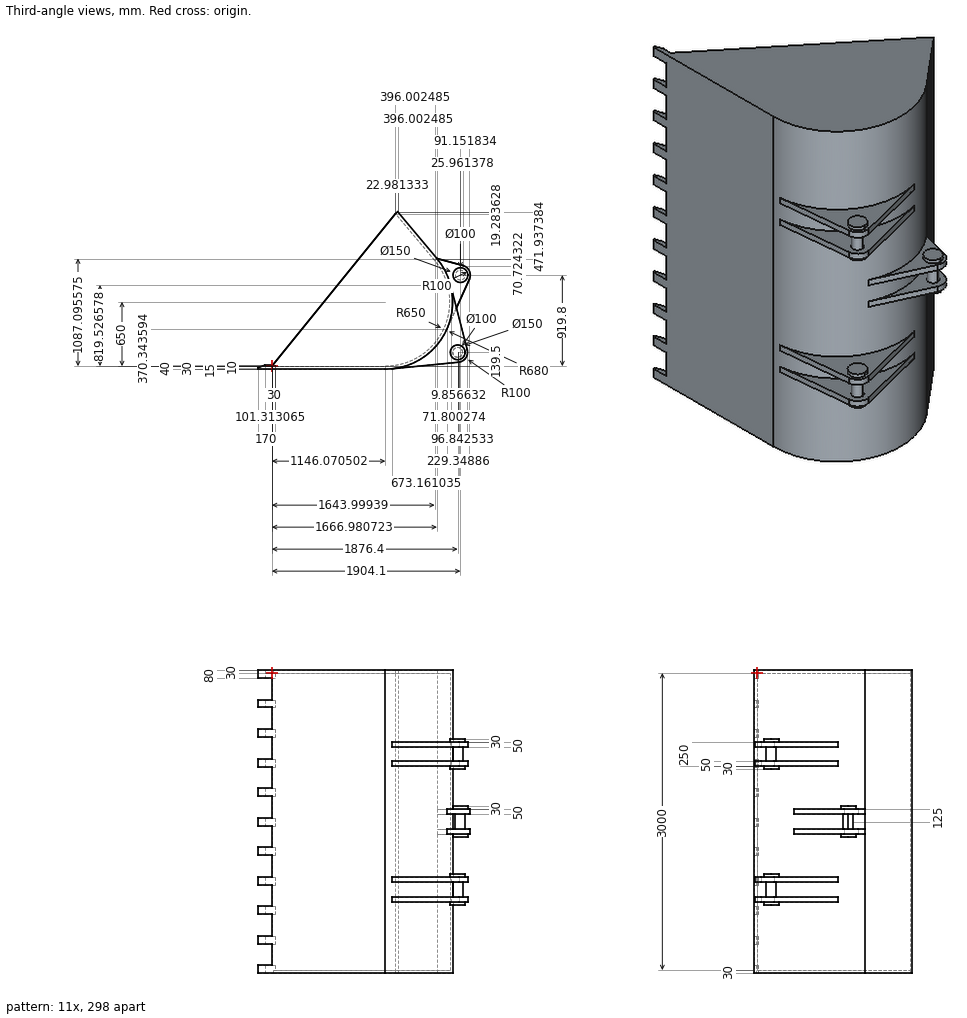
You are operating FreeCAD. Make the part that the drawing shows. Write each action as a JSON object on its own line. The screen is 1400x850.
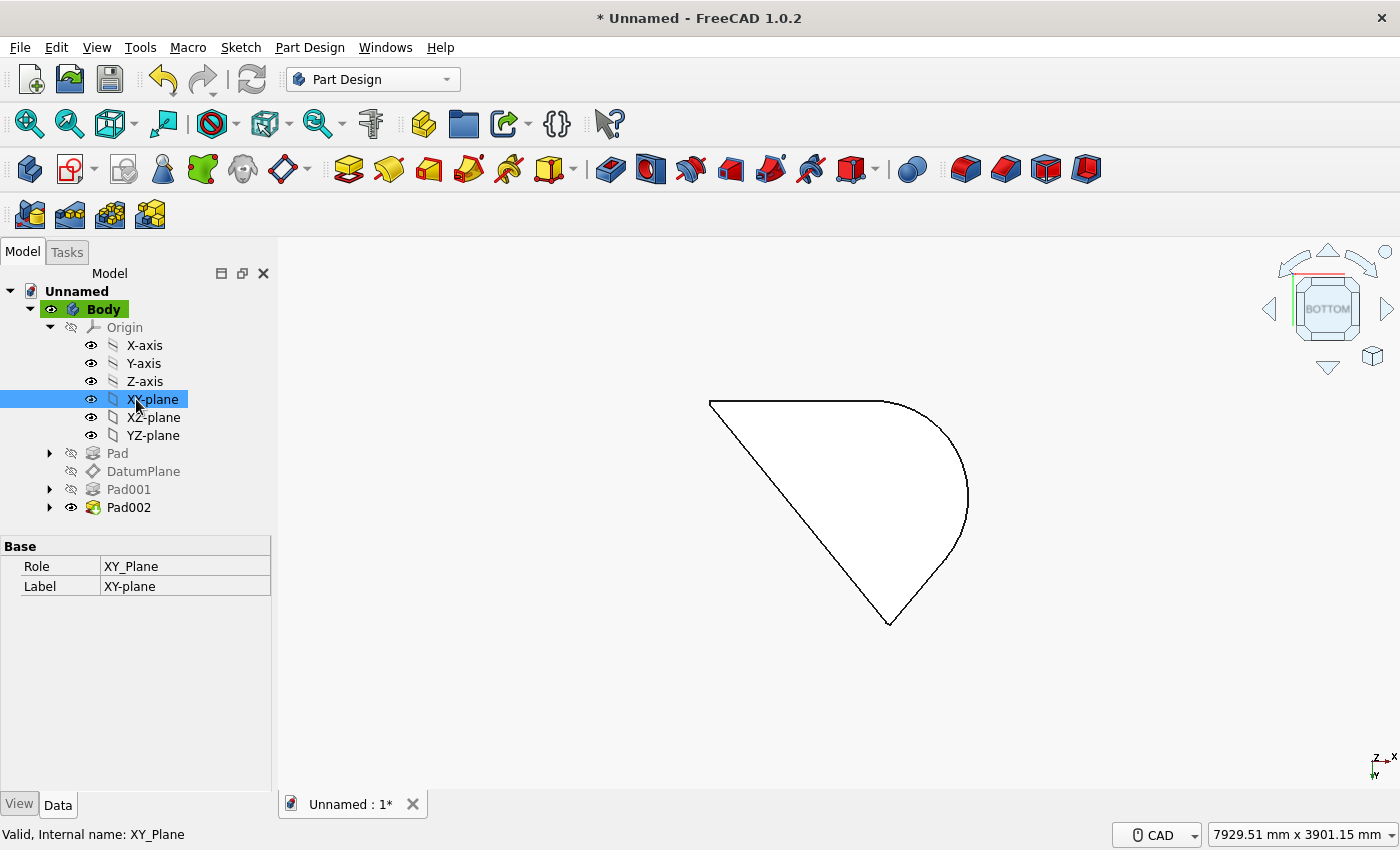
{"action": "left_click", "coordinate": [284, 170]}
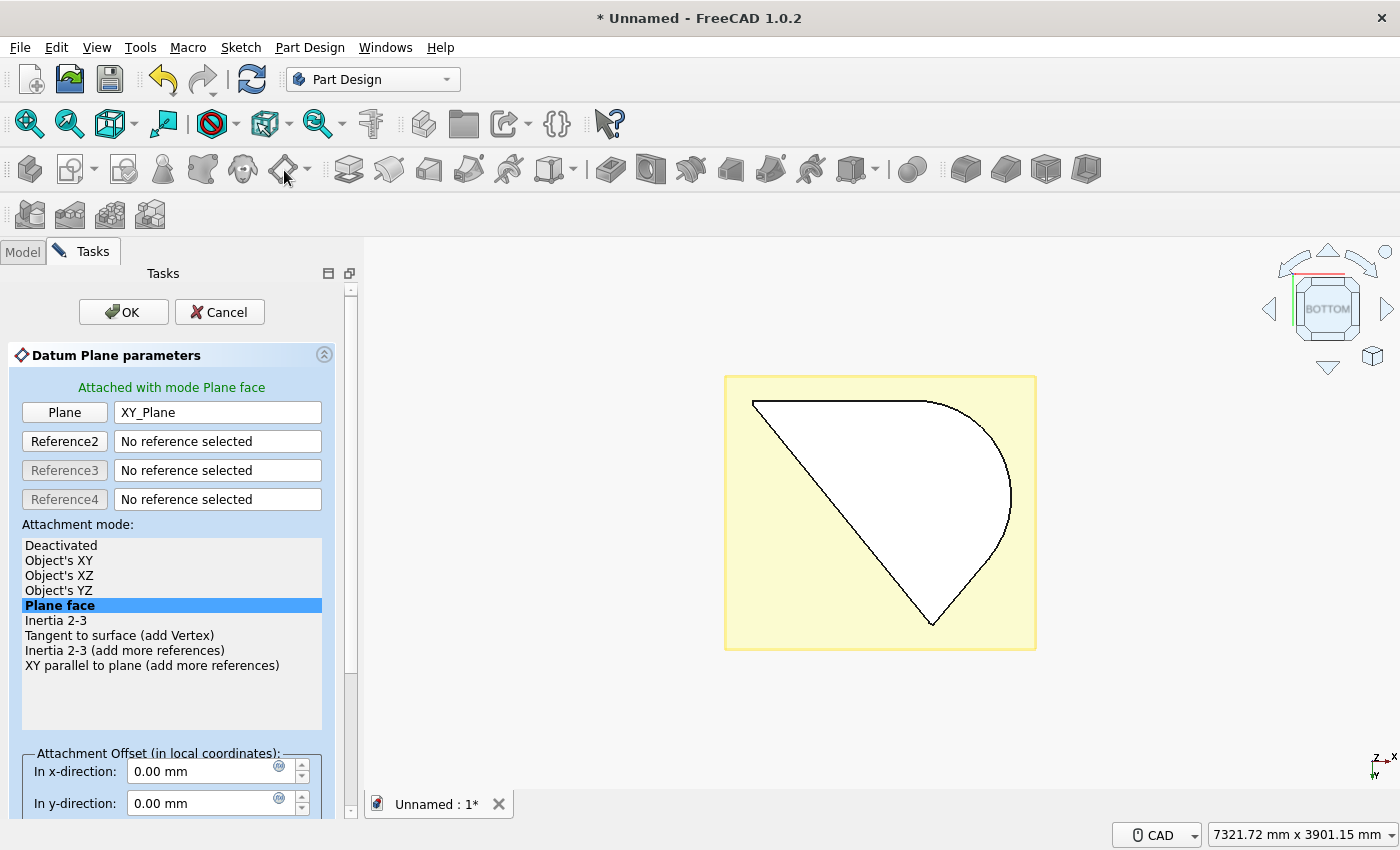
{"action": "scroll", "coordinate": [351, 550], "scroll_direction": "down", "scroll_amount": 2}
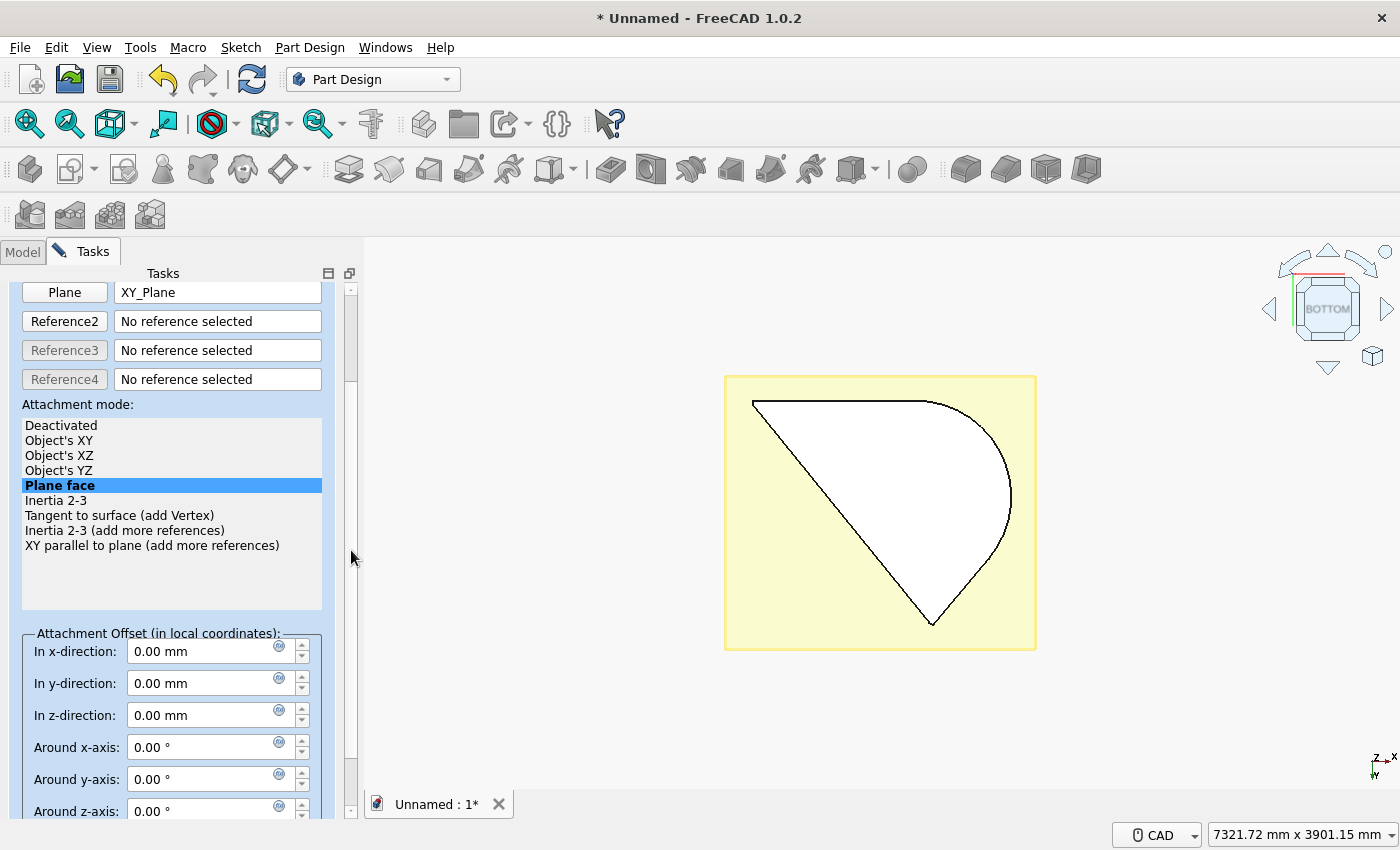
{"action": "triple_click", "coordinate": [210, 715]}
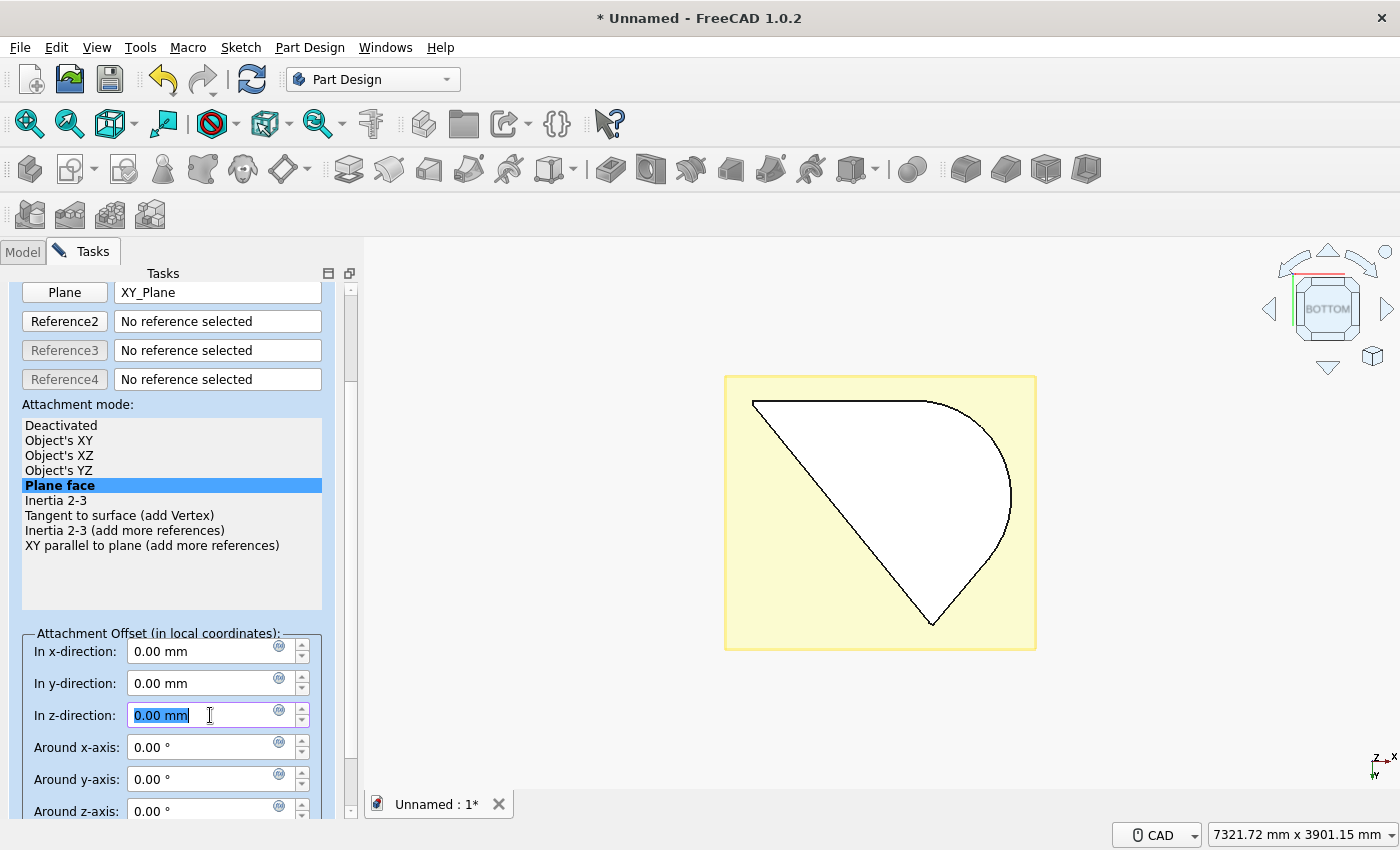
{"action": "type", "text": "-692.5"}
{"action": "key", "text": "Tab"}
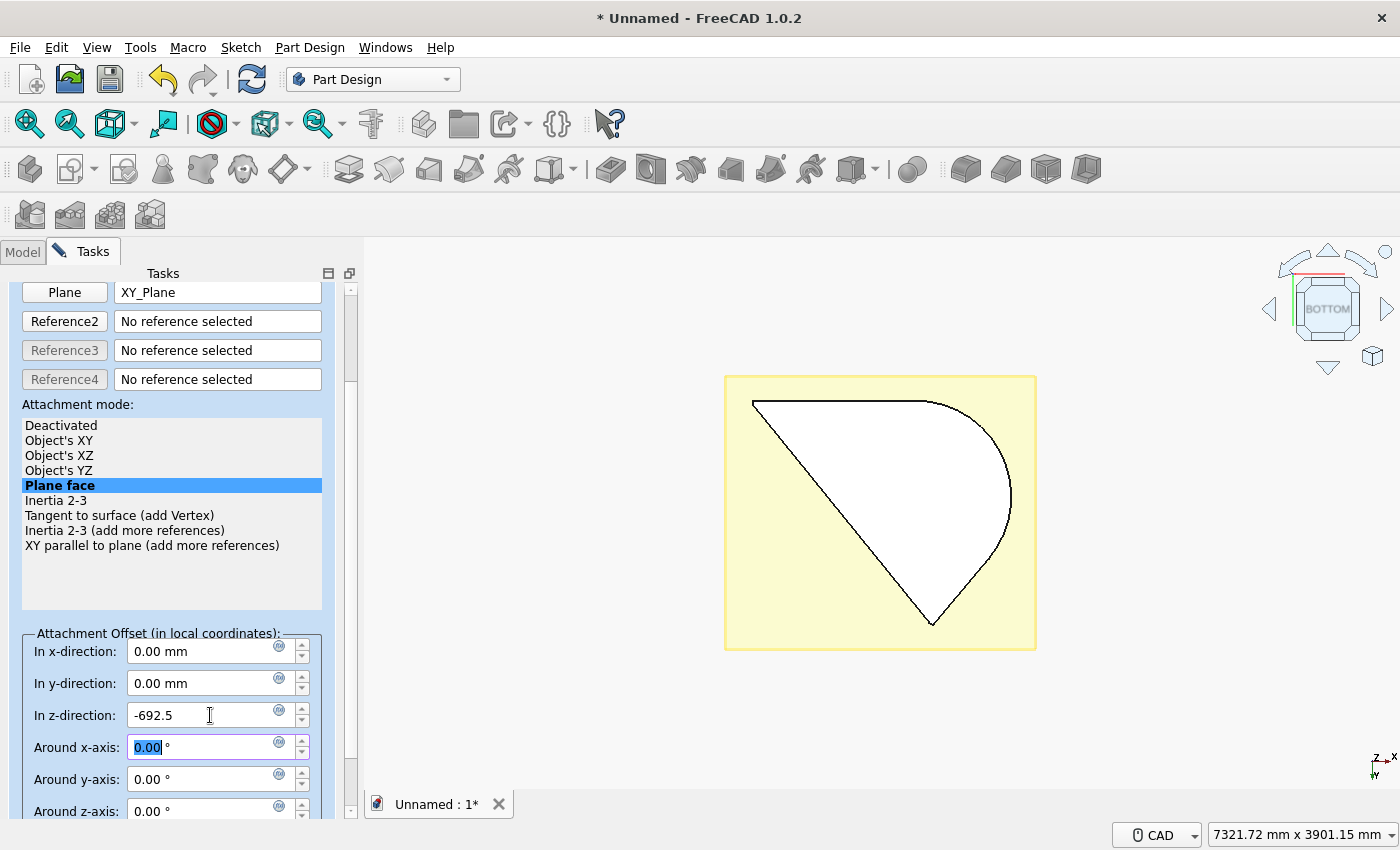
{"action": "scroll", "coordinate": [351, 550], "scroll_direction": "up", "scroll_amount": 3}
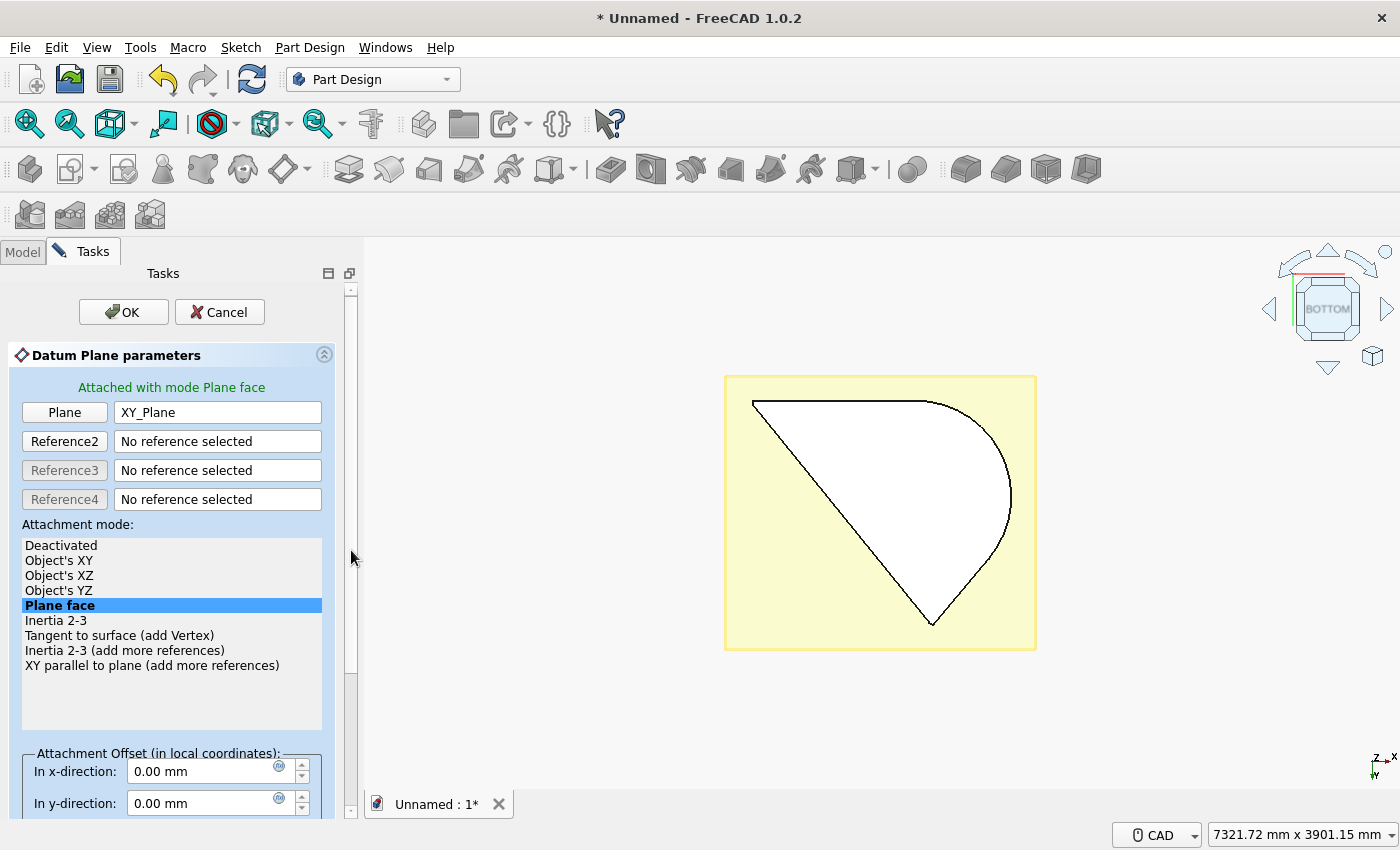
{"action": "left_click", "coordinate": [124, 312]}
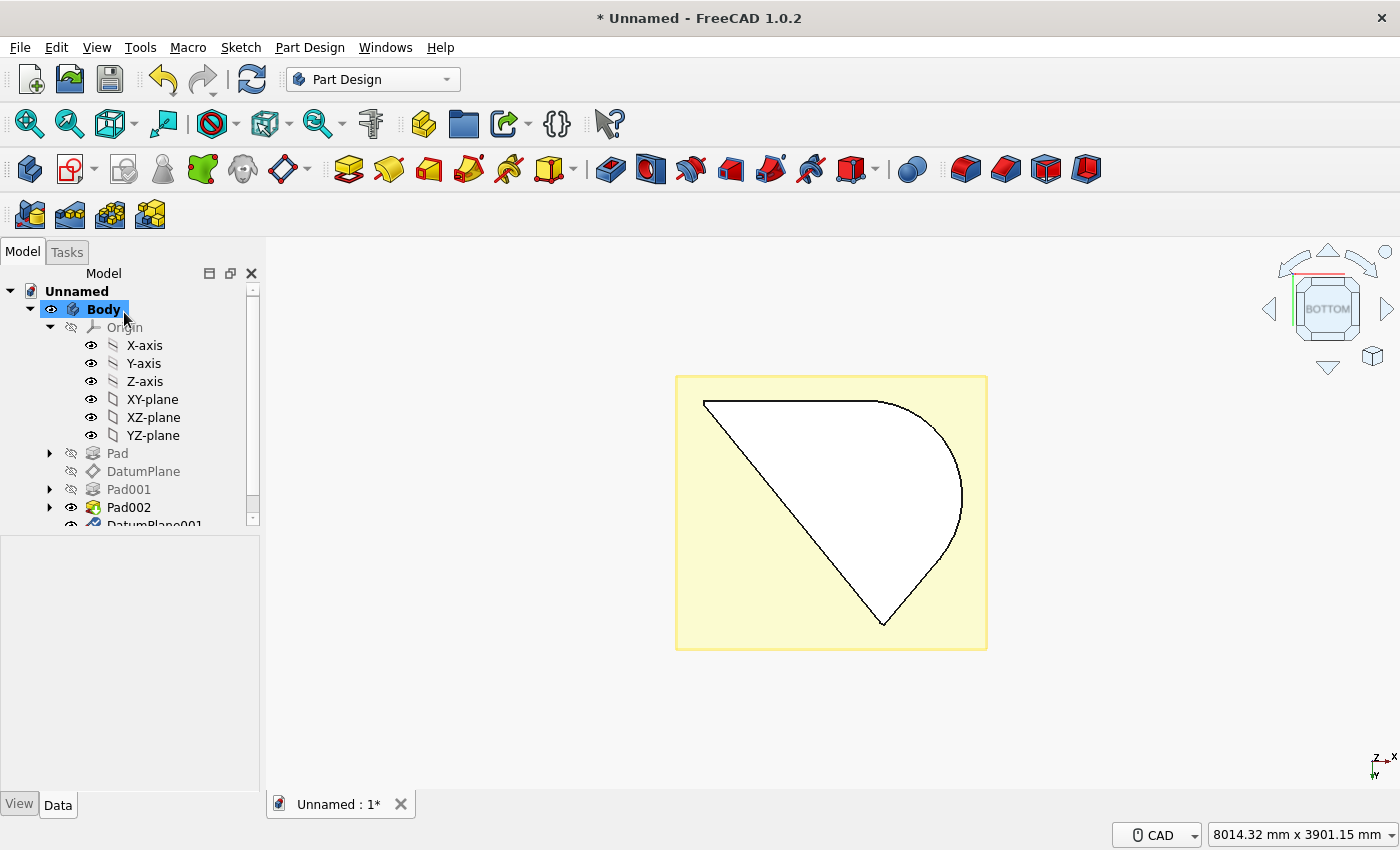
{"action": "left_click", "coordinate": [116, 525]}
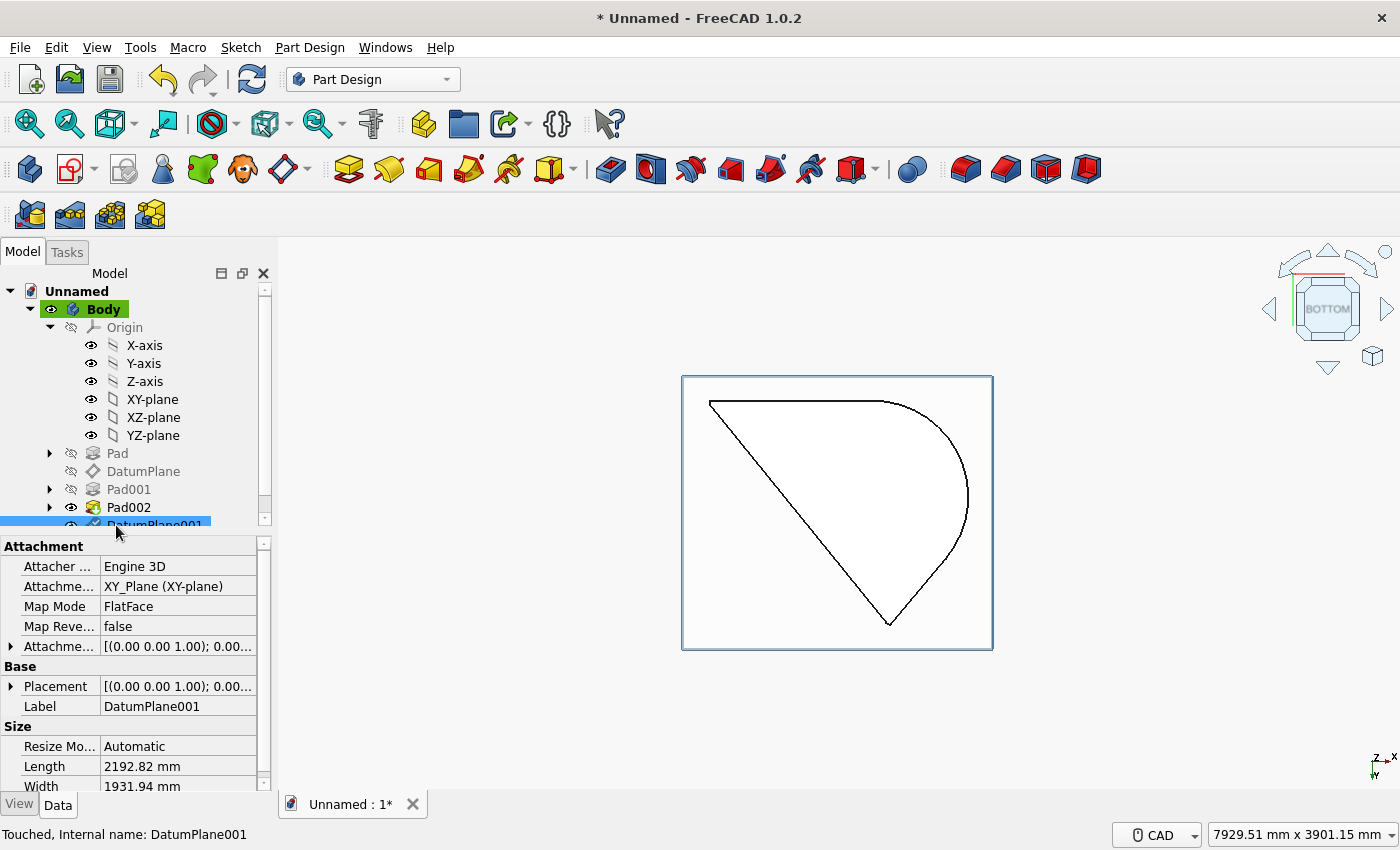
{"action": "left_click", "coordinate": [70, 170]}